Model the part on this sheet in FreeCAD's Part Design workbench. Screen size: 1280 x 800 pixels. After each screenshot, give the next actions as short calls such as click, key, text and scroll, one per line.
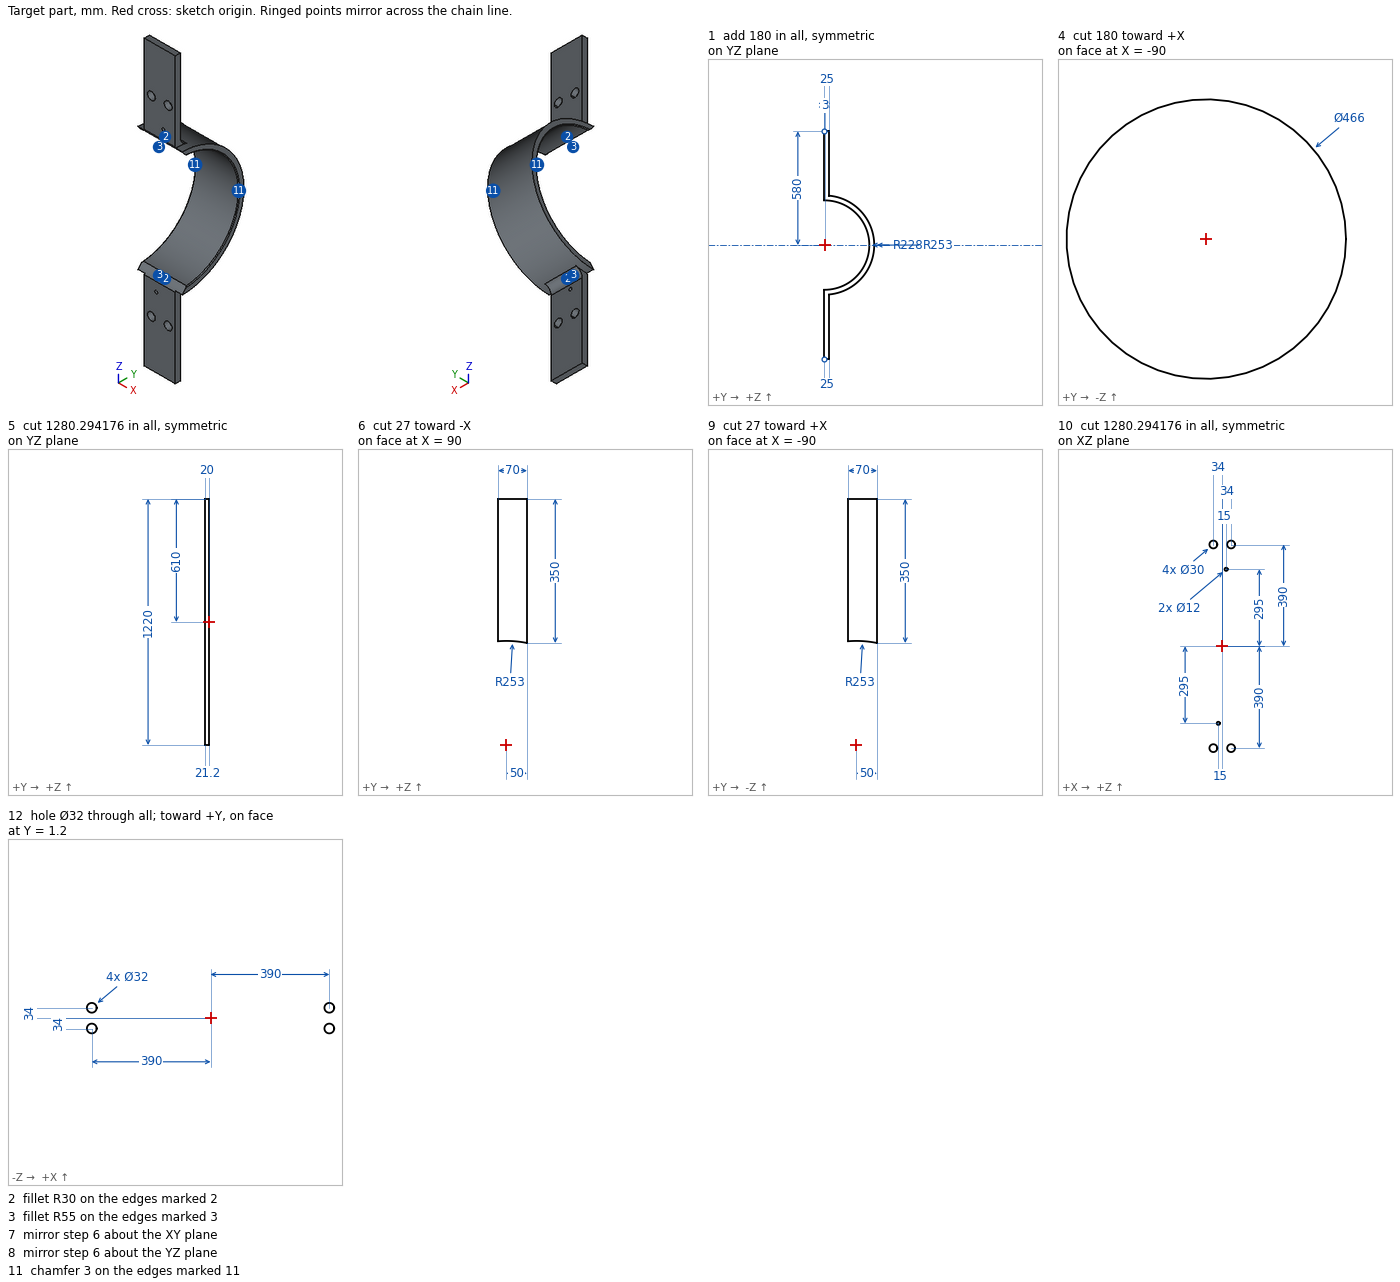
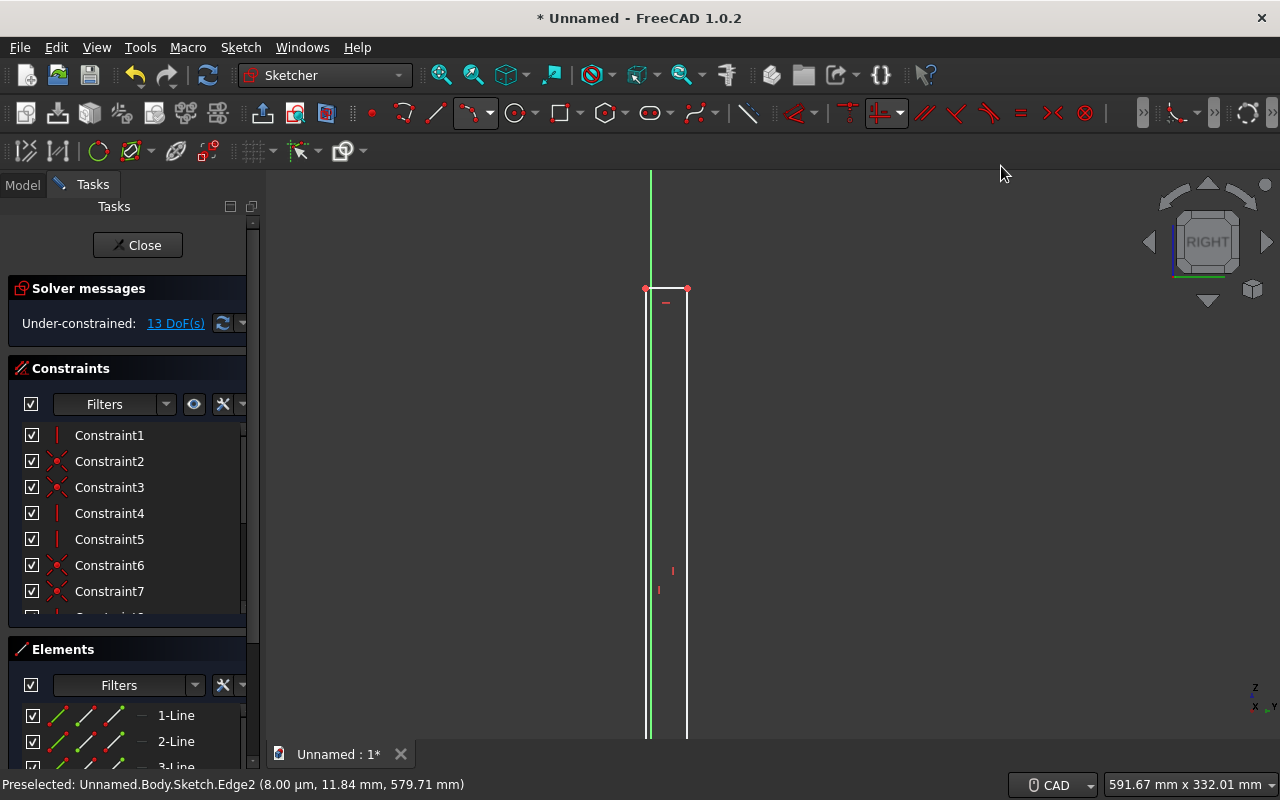
scroll(673, 291, down, 9)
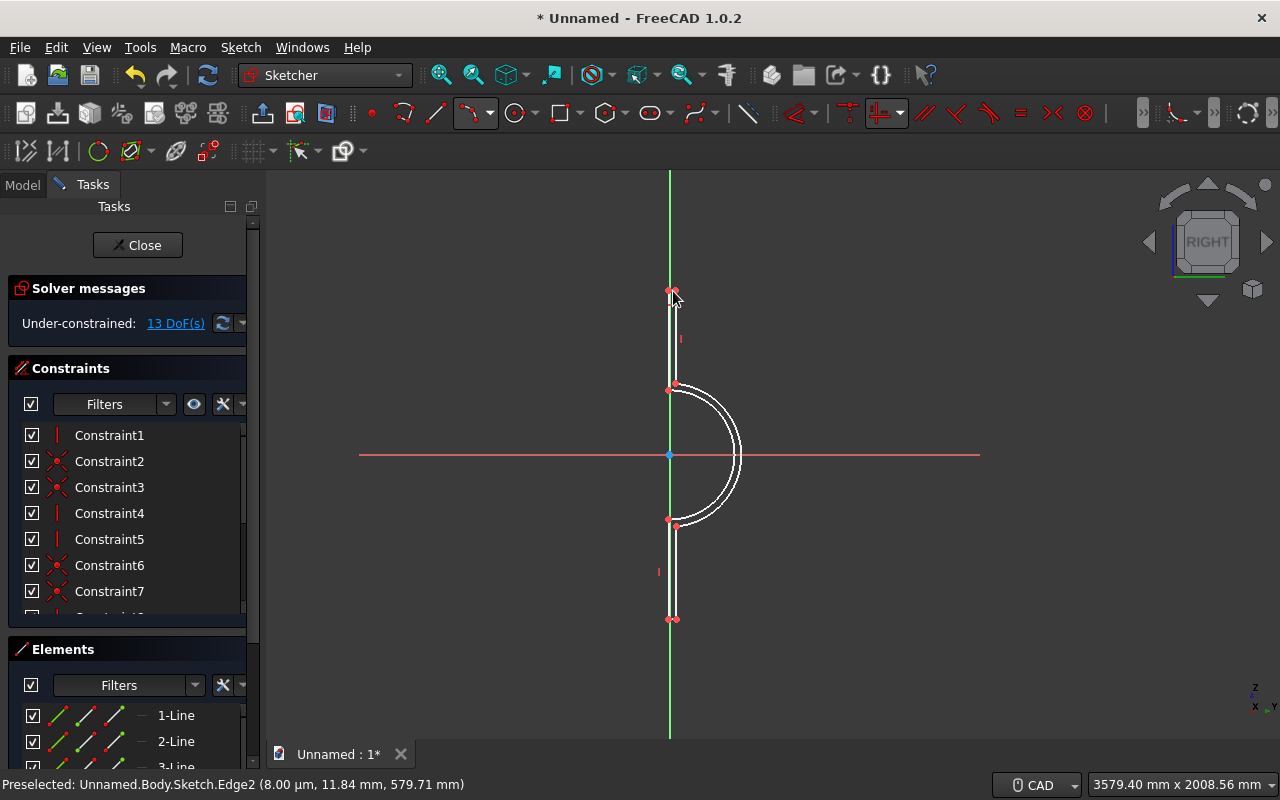
scroll(674, 620, up, 10)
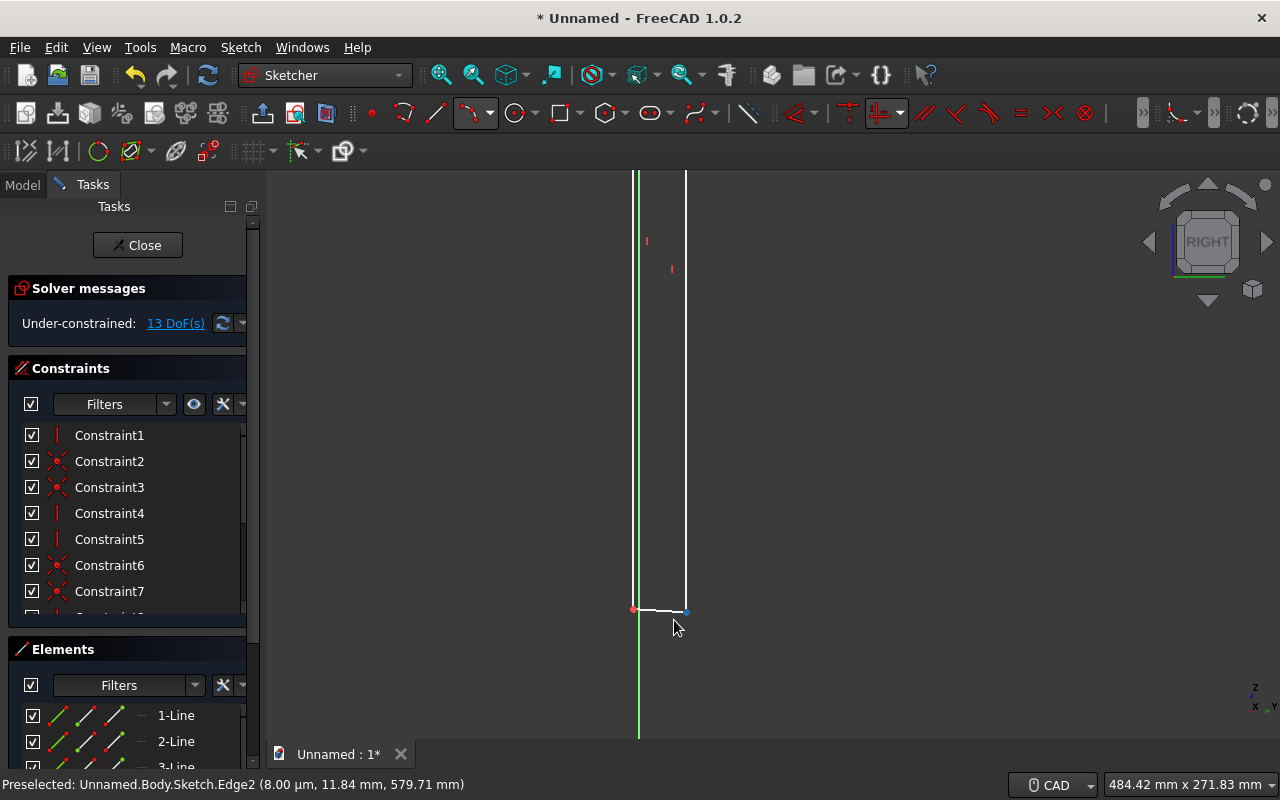
click(670, 611)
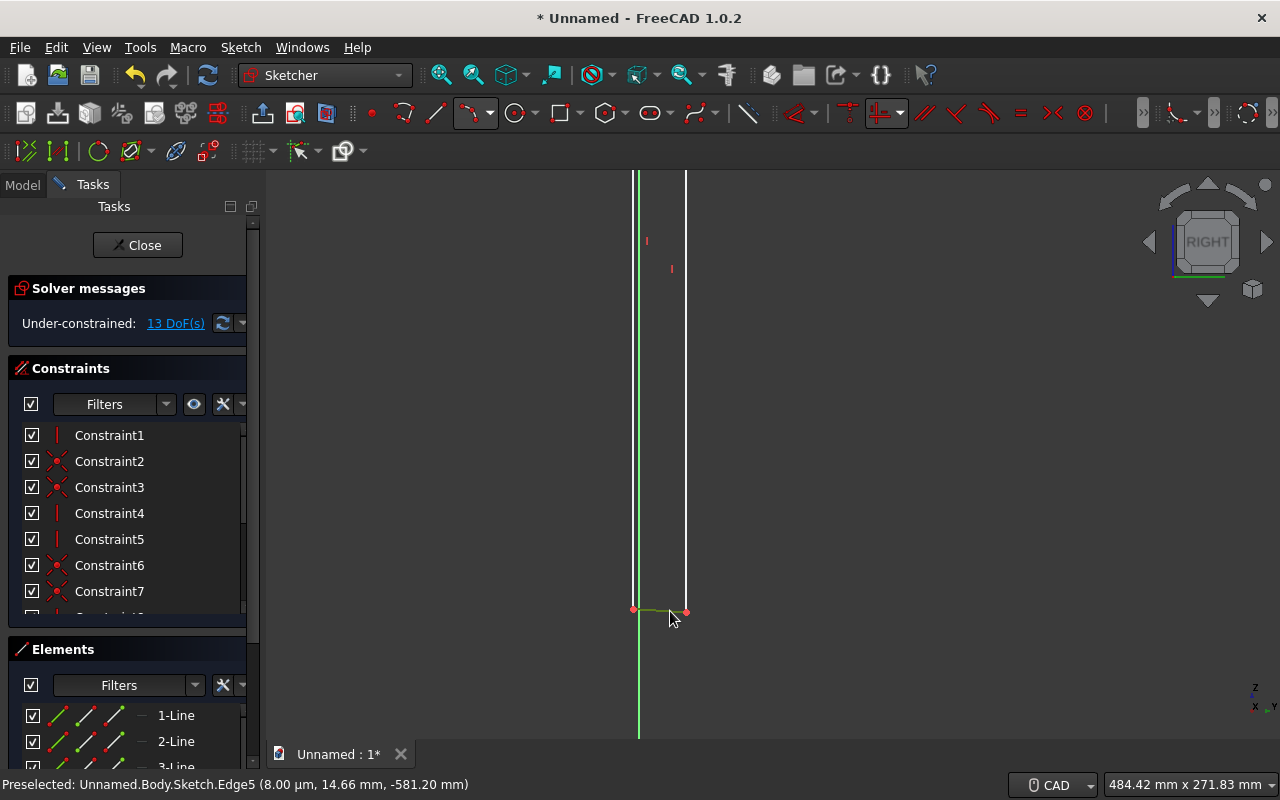
key(h)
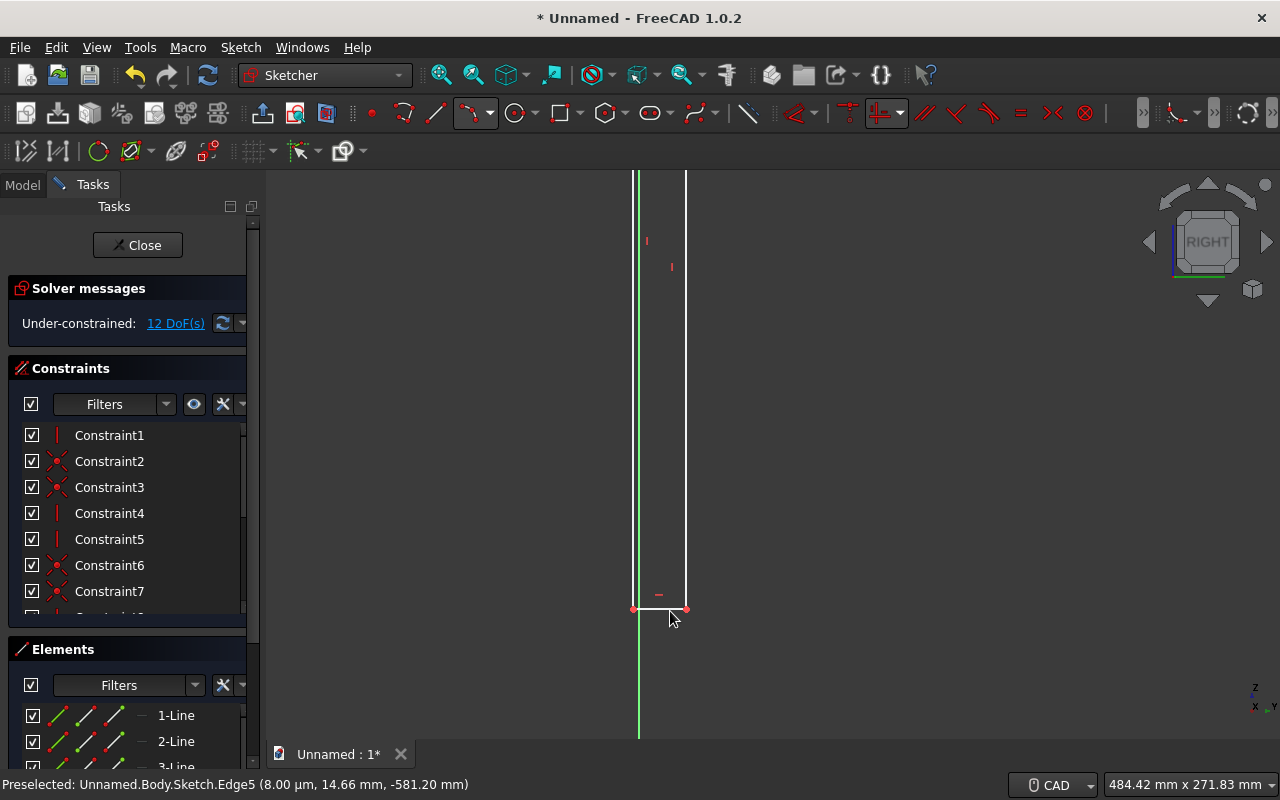
scroll(674, 620, down, 10)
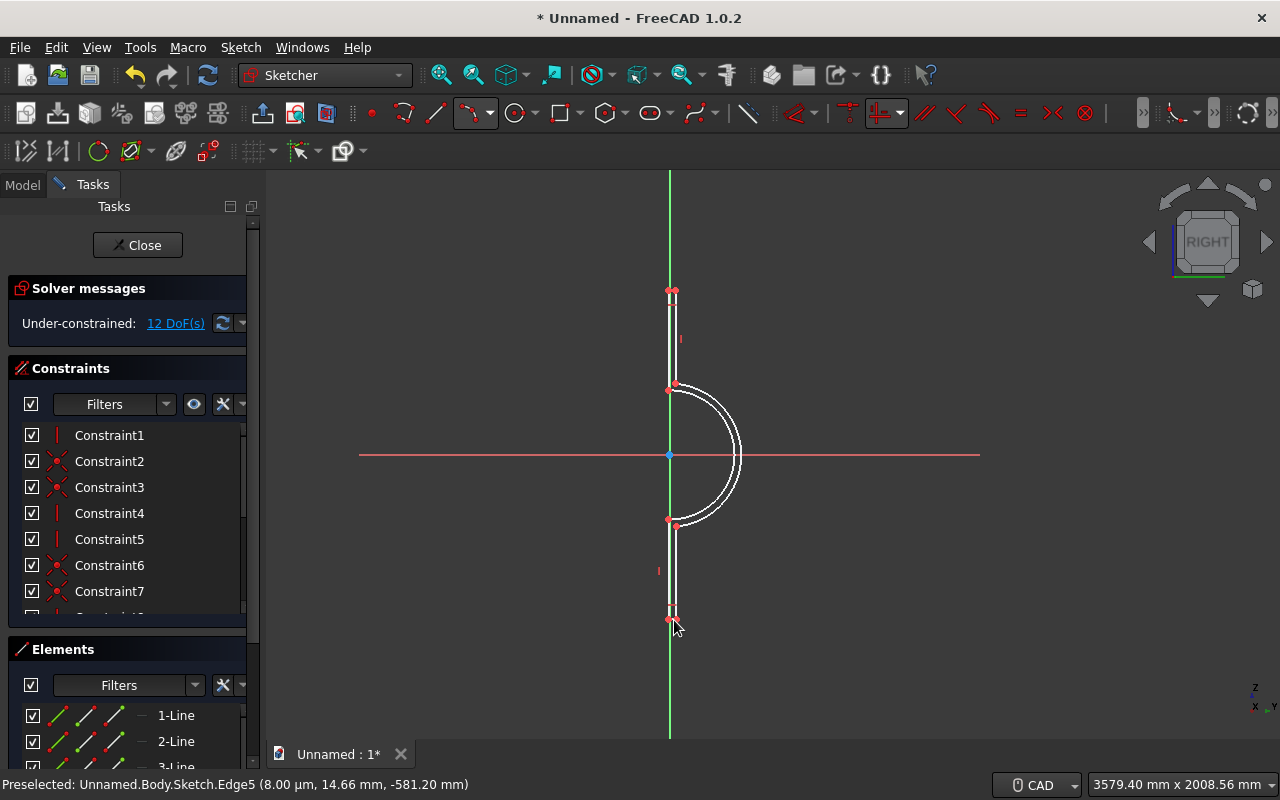
scroll(722, 493, up, 4)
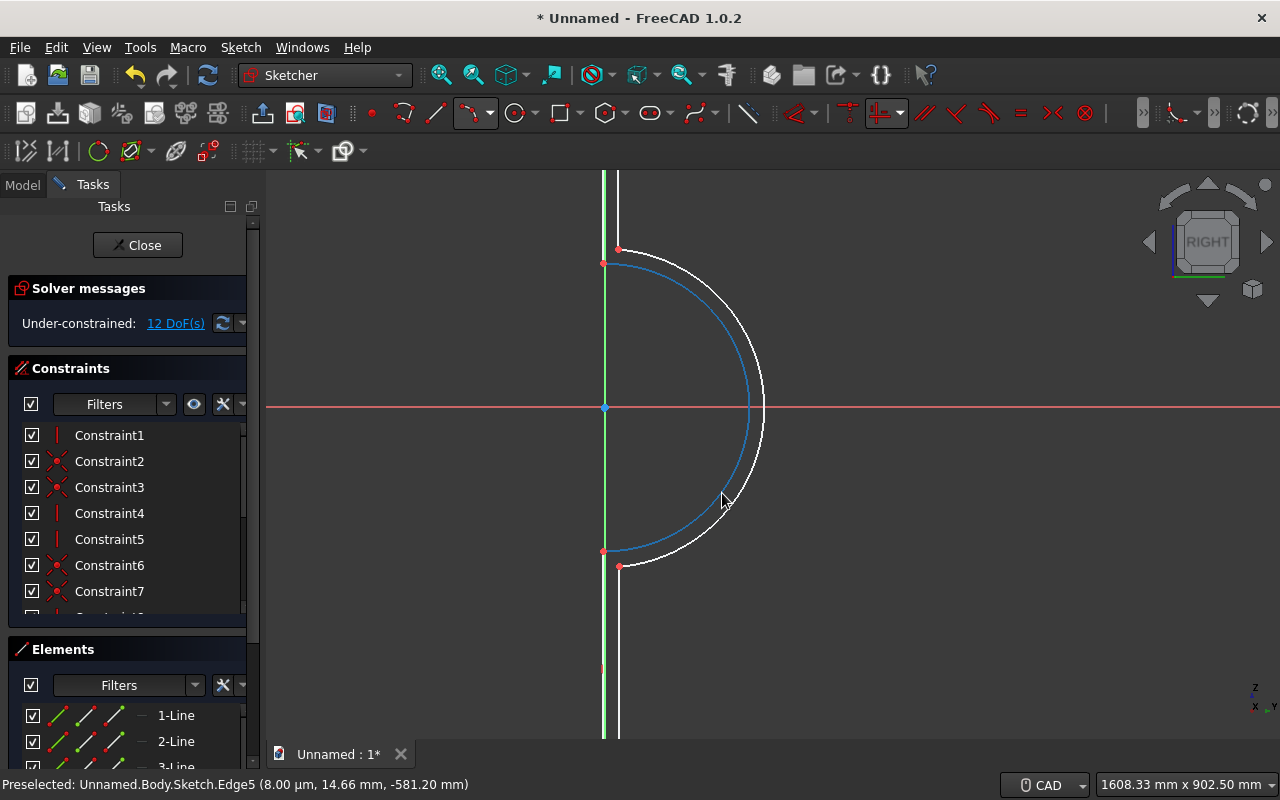
click(721, 493)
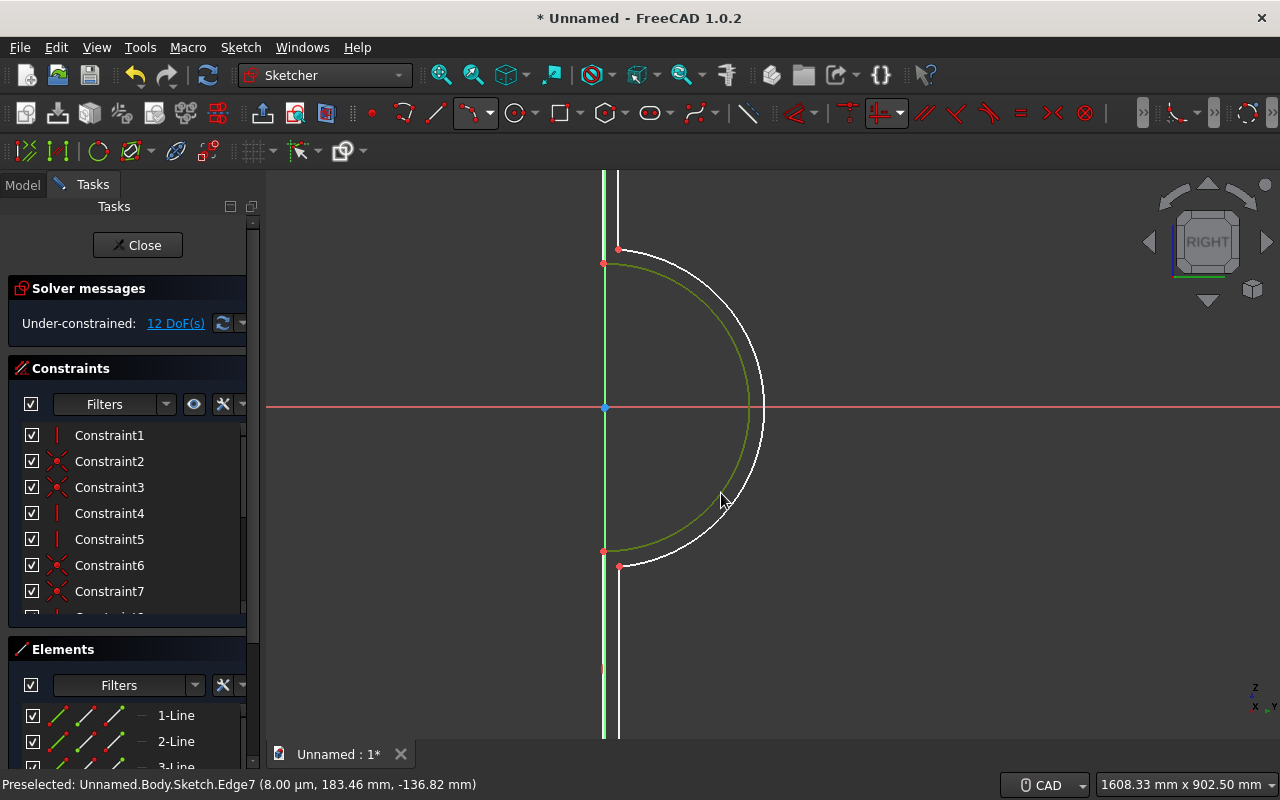
click(737, 497)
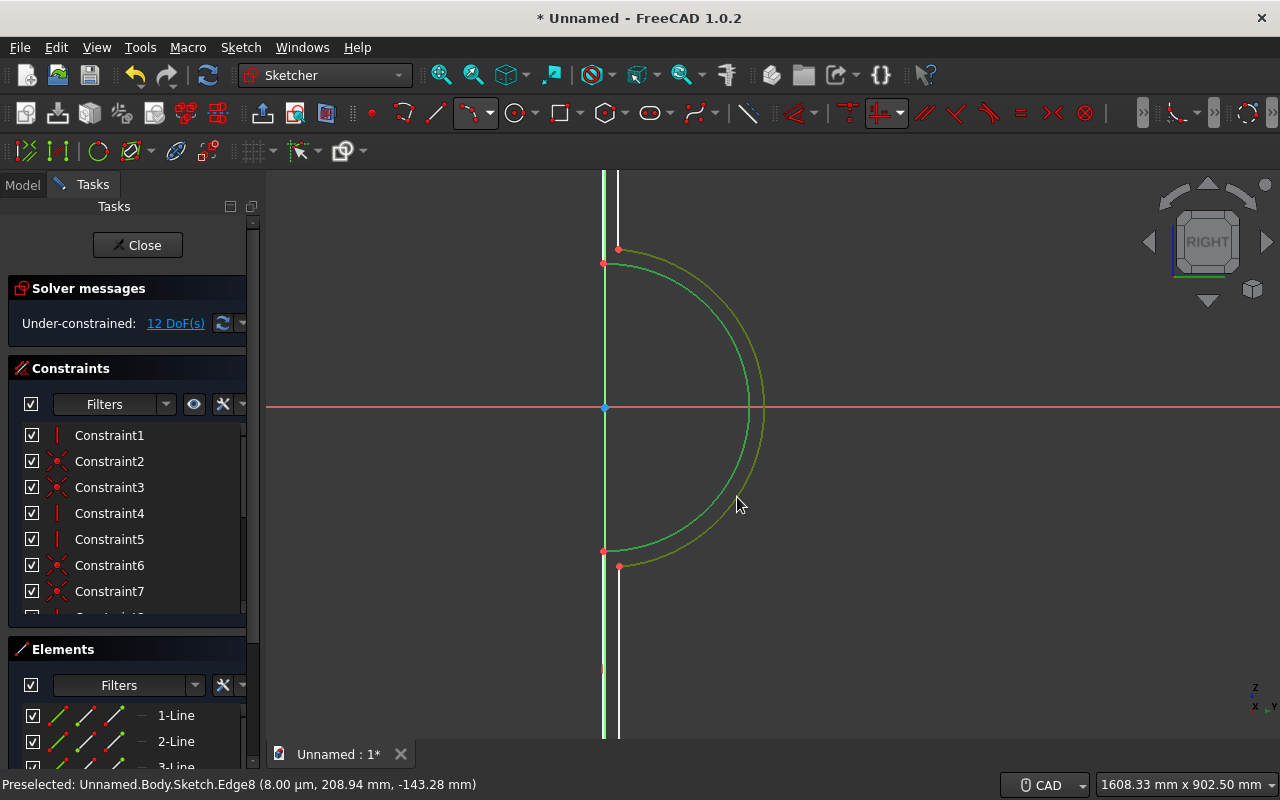
click(848, 114)